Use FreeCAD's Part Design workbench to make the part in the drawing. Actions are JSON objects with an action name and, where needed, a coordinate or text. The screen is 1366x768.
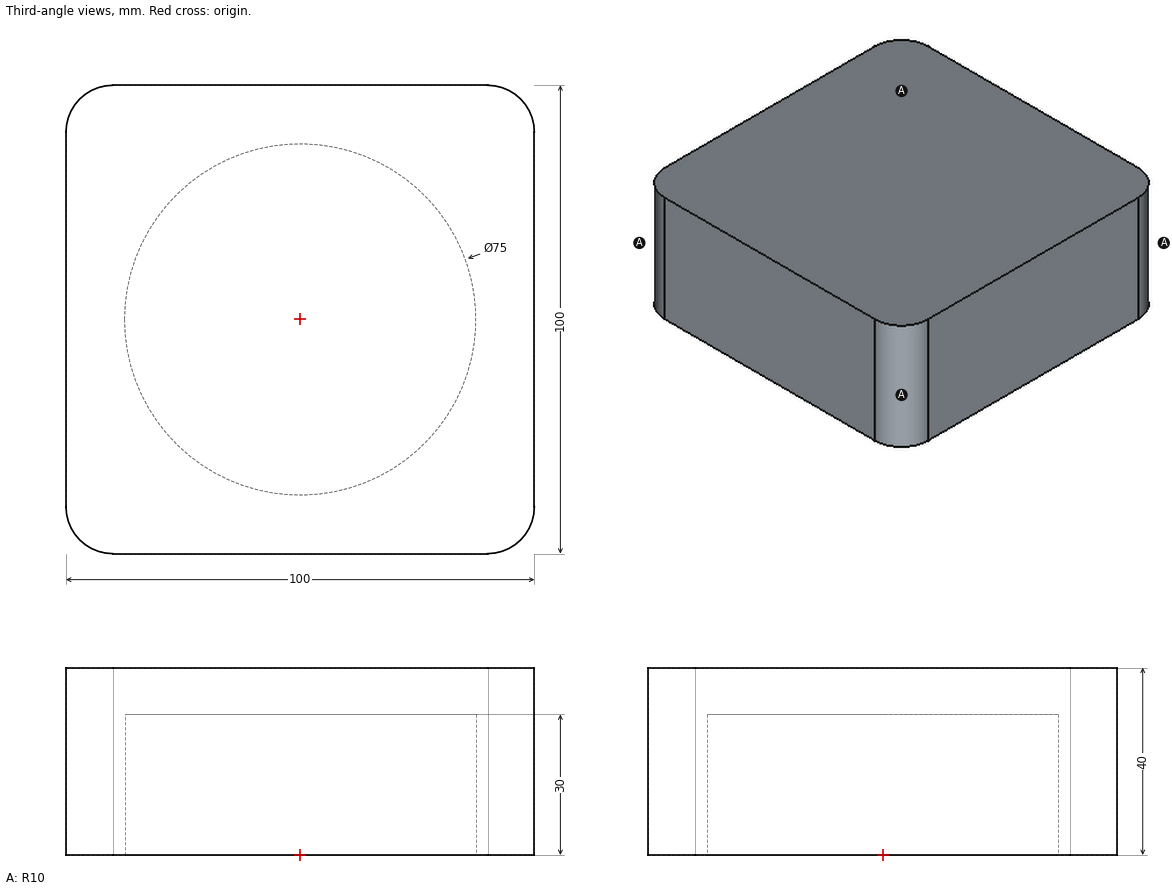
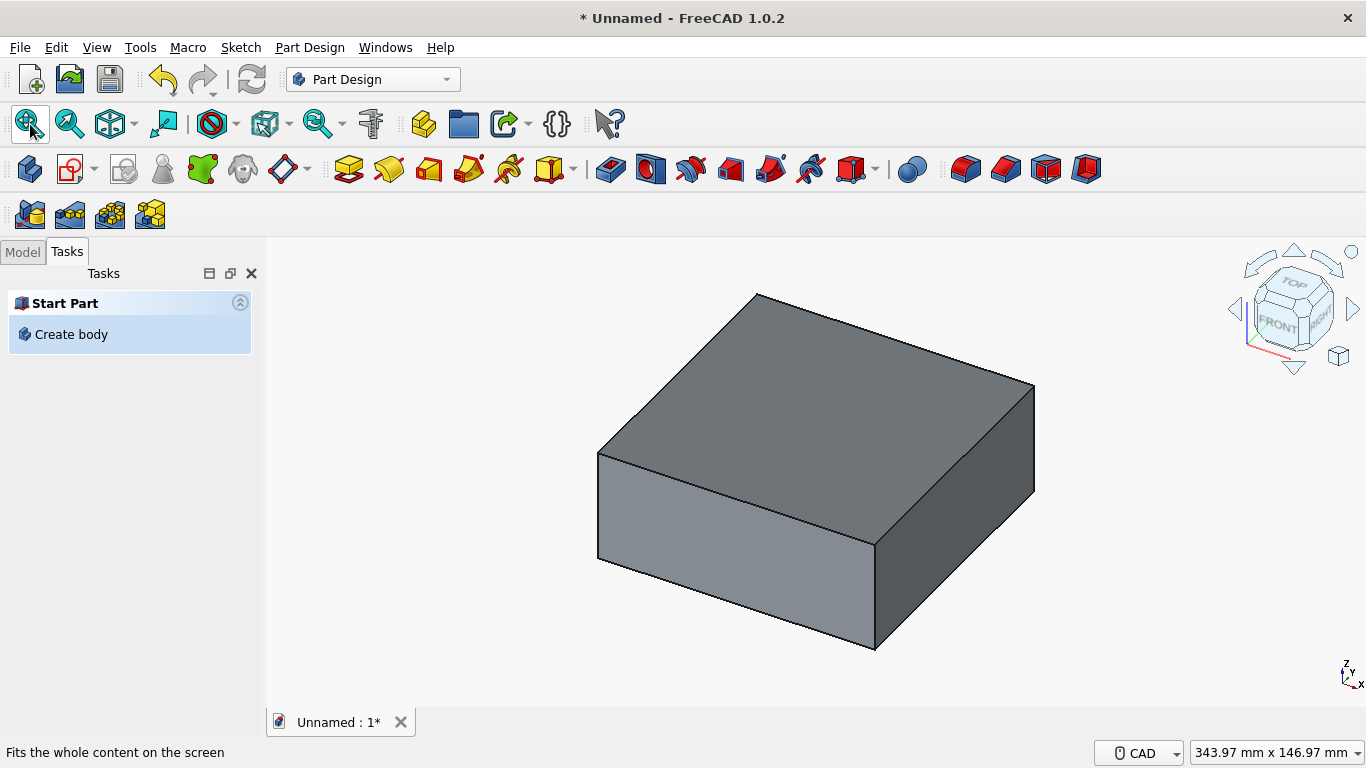
{"action": "left_click", "coordinate": [70, 170]}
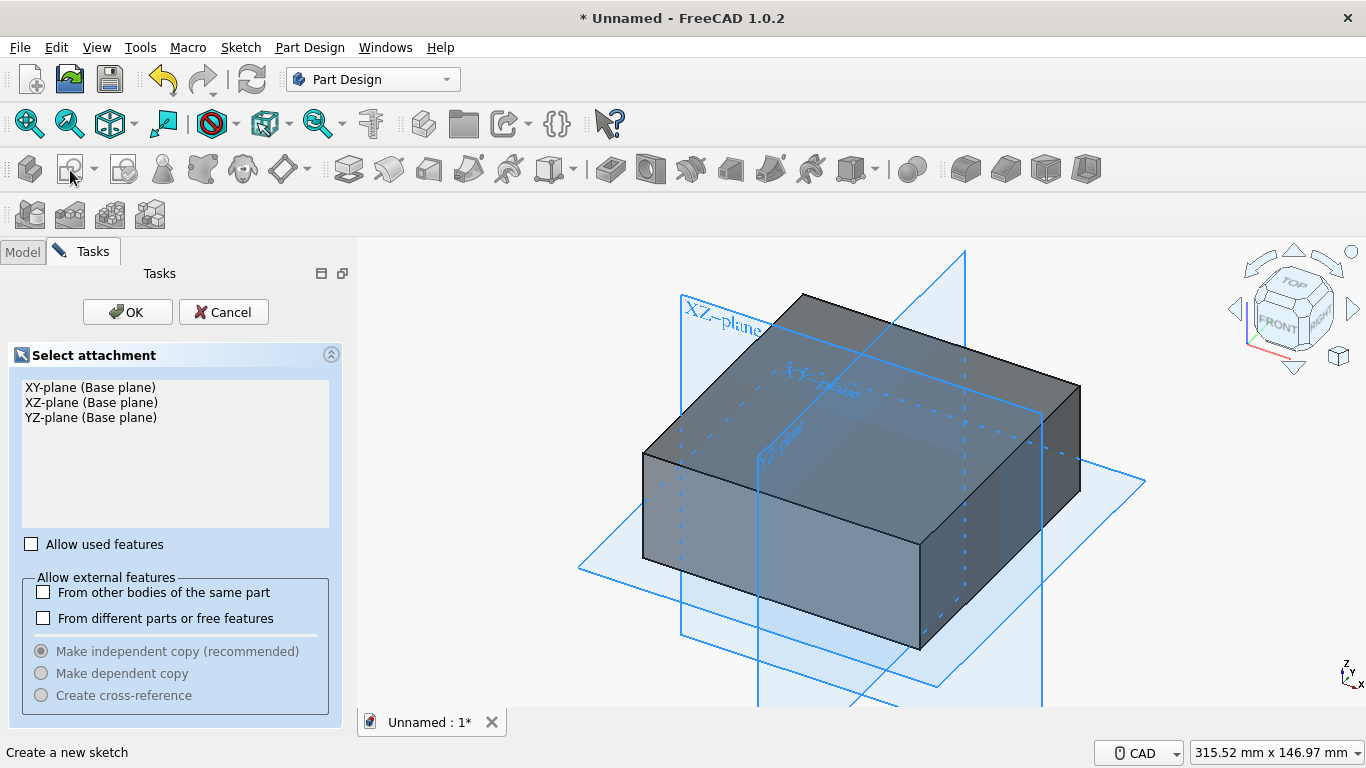
{"action": "left_click", "coordinate": [82, 388]}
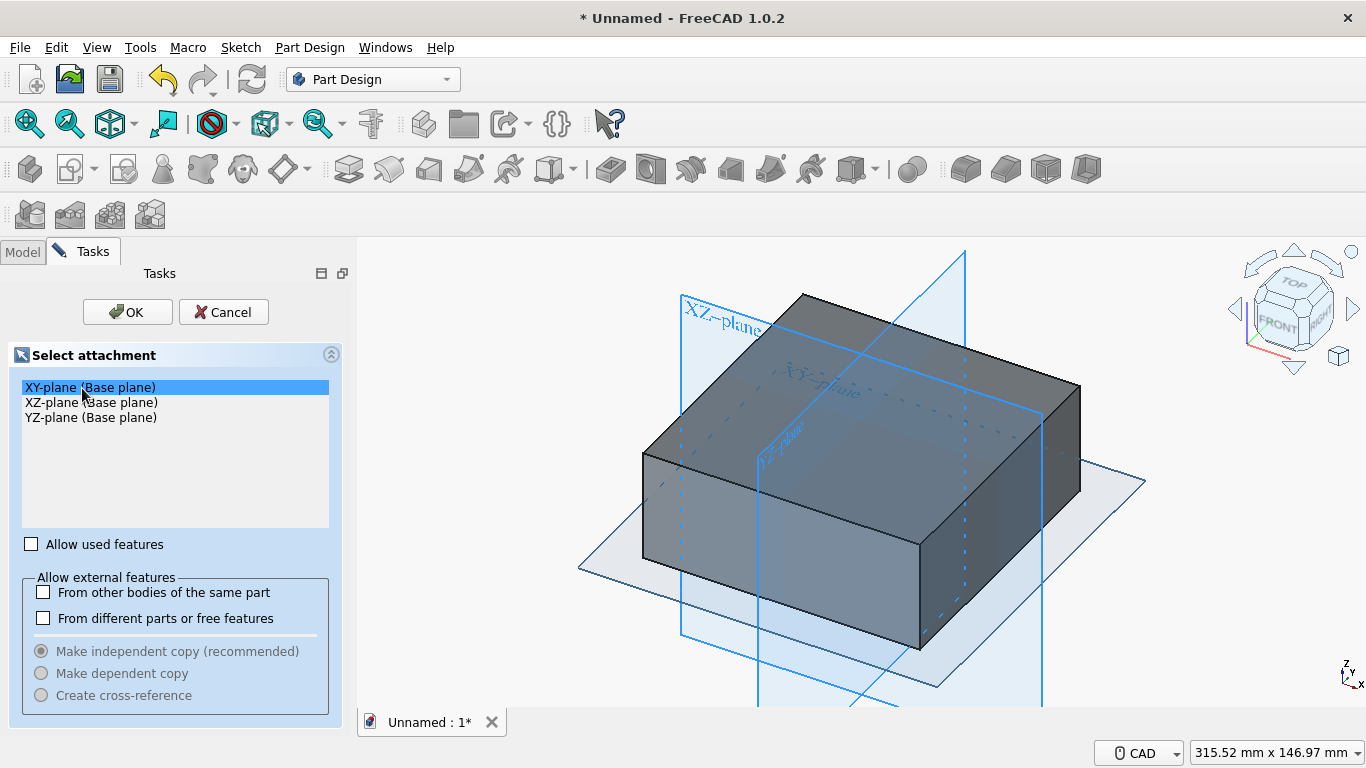
{"action": "left_click", "coordinate": [128, 312]}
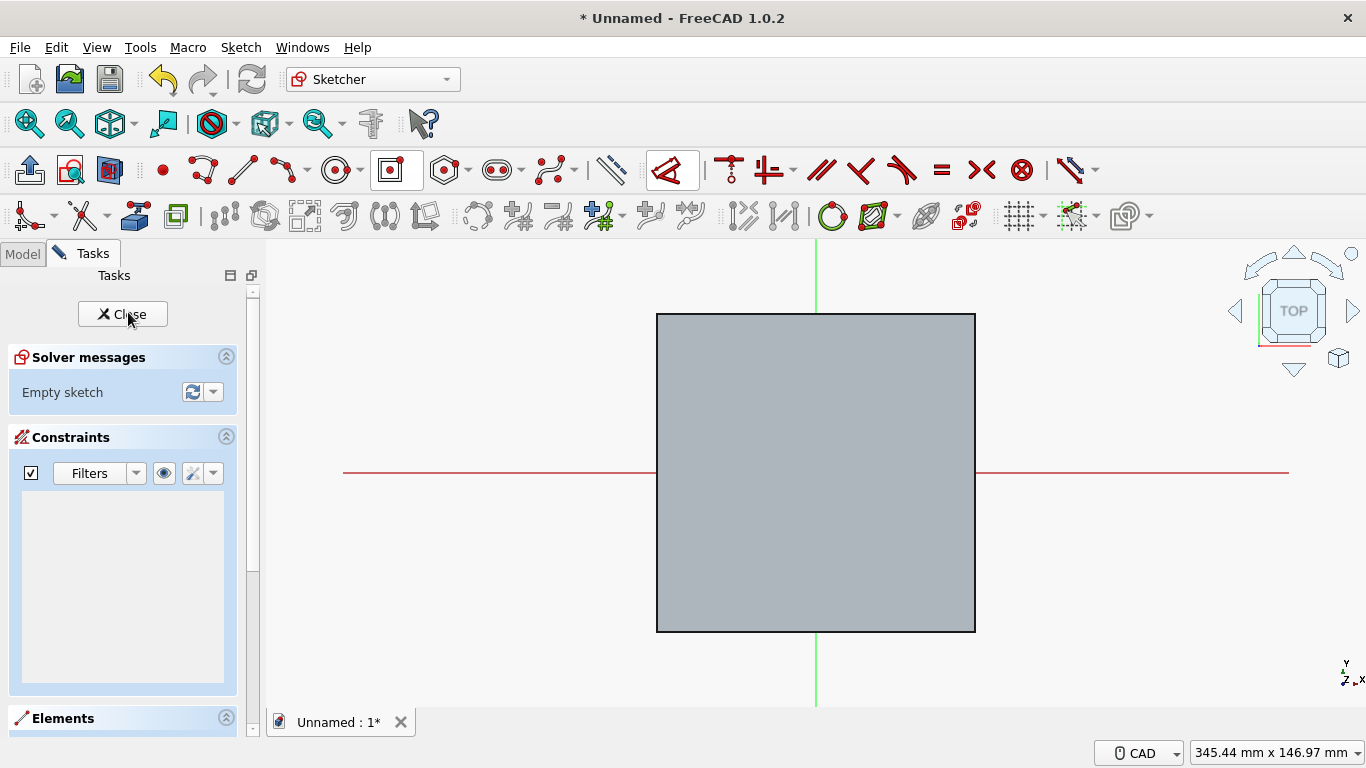
{"action": "left_click", "coordinate": [110, 170]}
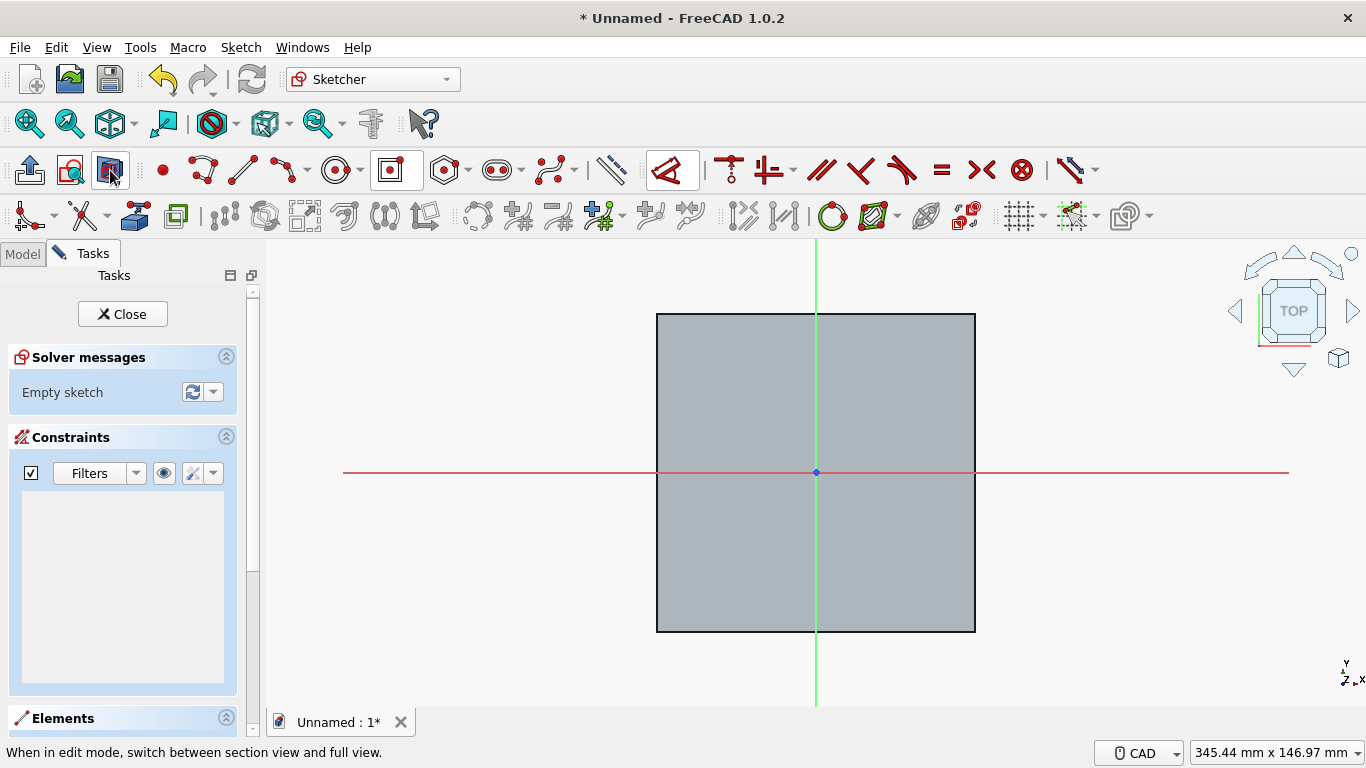
{"action": "key", "text": "g c"}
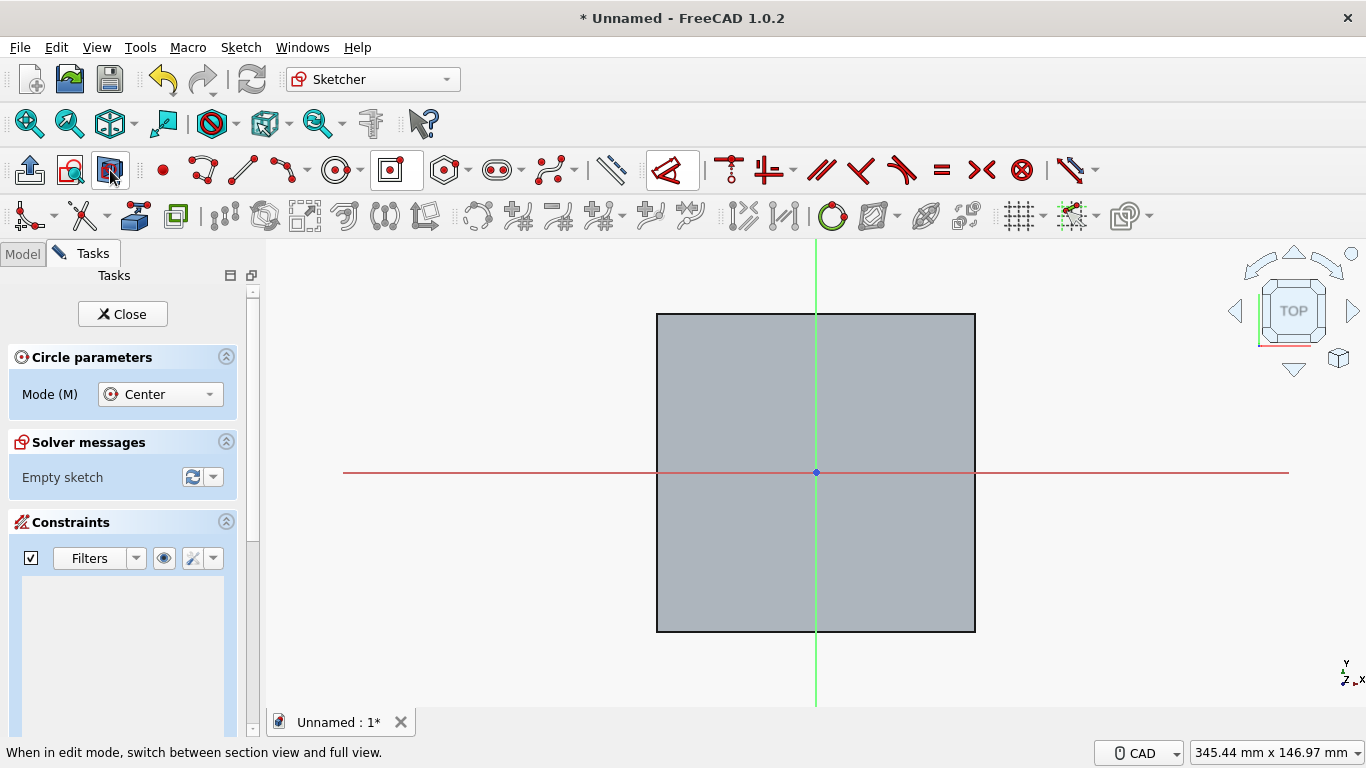
{"action": "left_click", "coordinate": [816, 473]}
{"action": "left_click", "coordinate": [900, 389]}
{"action": "key", "text": "Escape"}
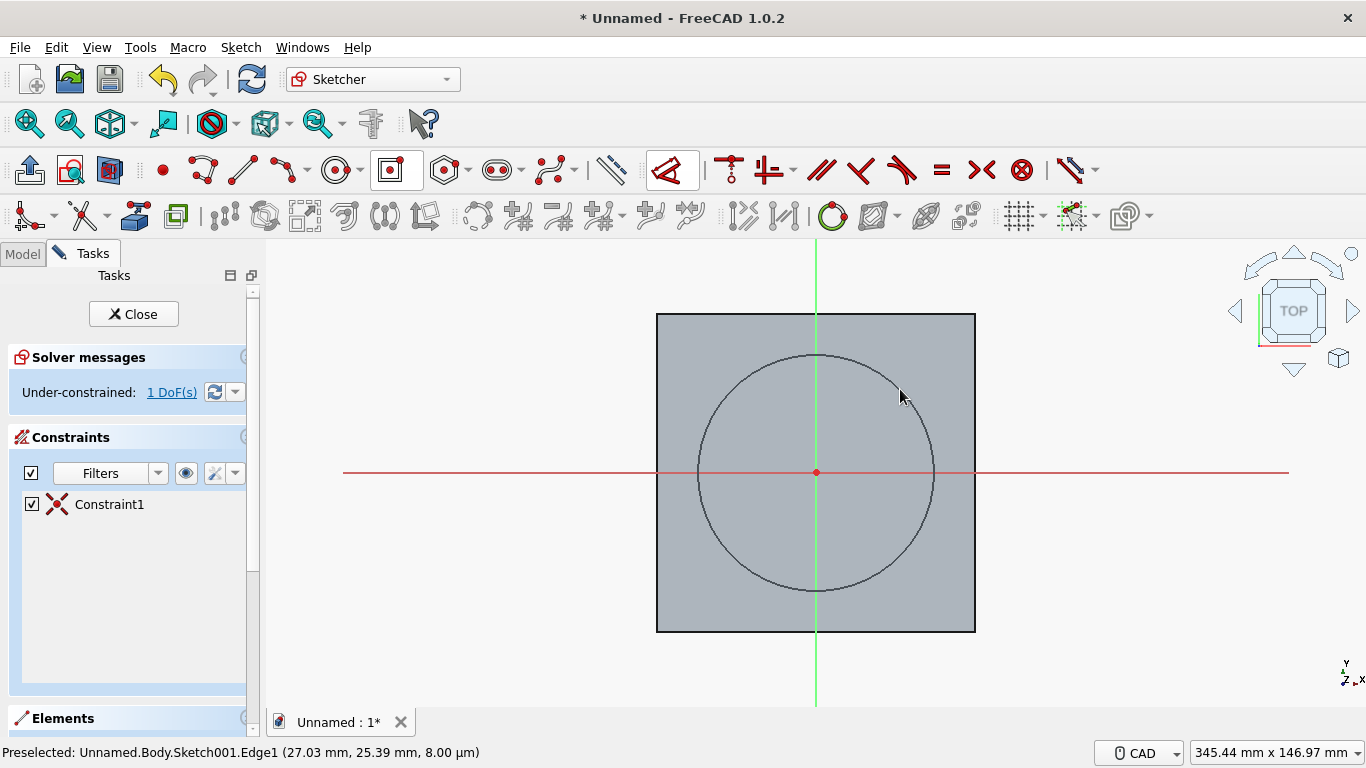
{"action": "key", "text": "d"}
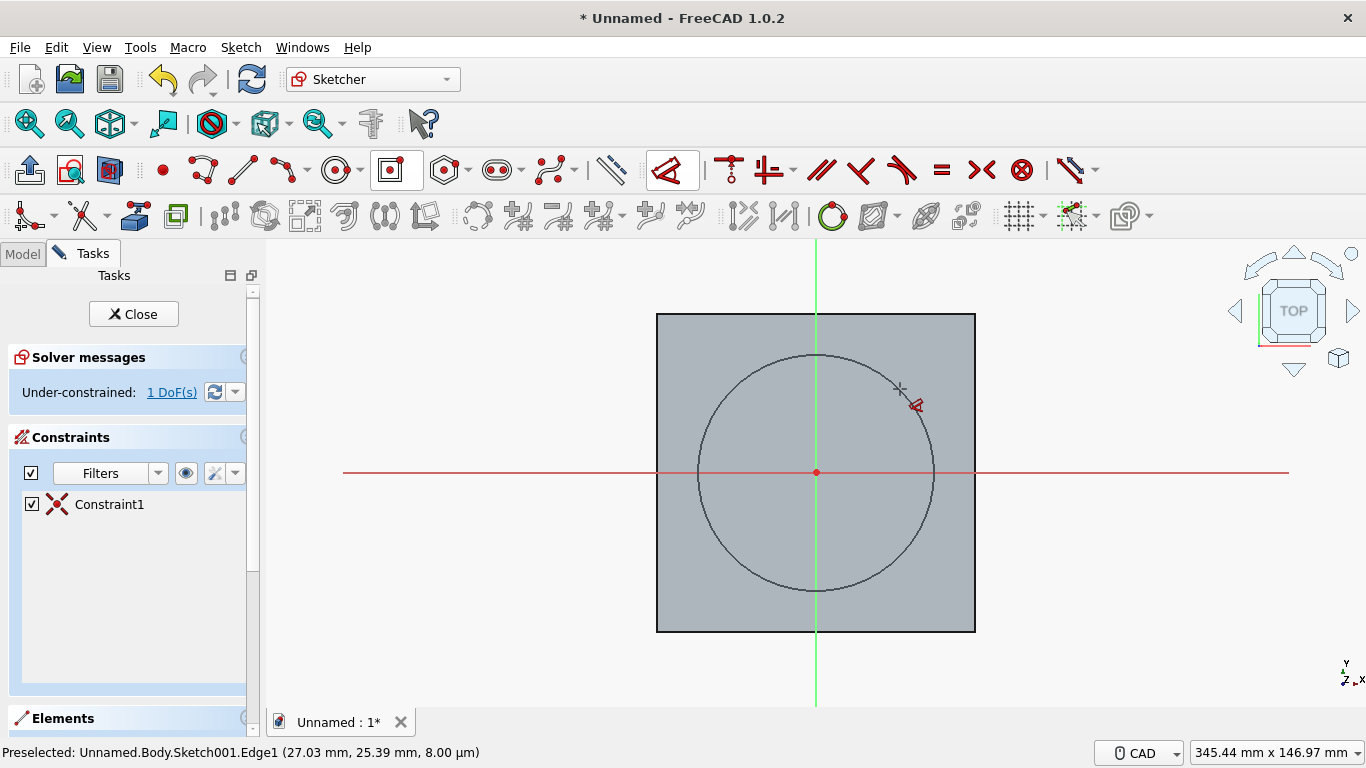
{"action": "left_click", "coordinate": [899, 389]}
{"action": "left_click", "coordinate": [921, 366]}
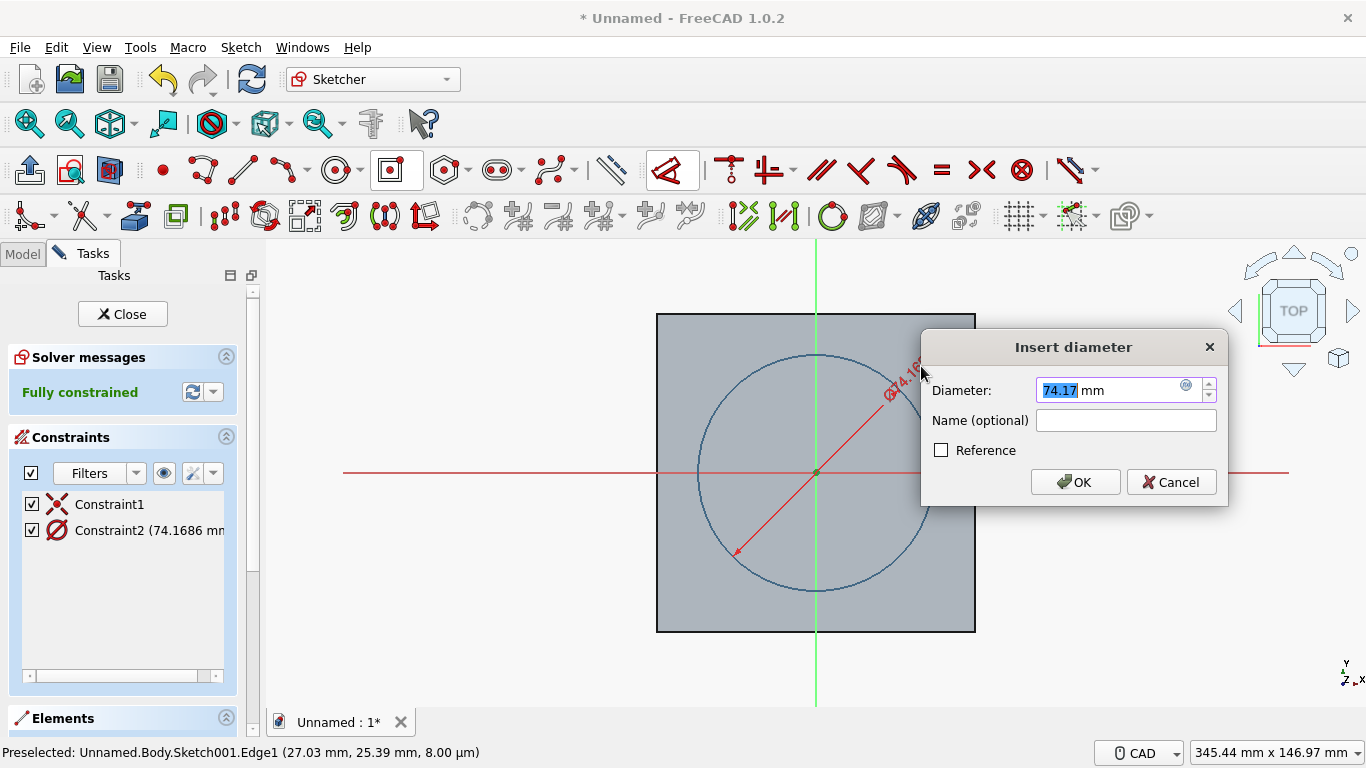
{"action": "type", "text": "75"}
{"action": "key", "text": "Return"}
{"action": "key", "text": "Escape"}